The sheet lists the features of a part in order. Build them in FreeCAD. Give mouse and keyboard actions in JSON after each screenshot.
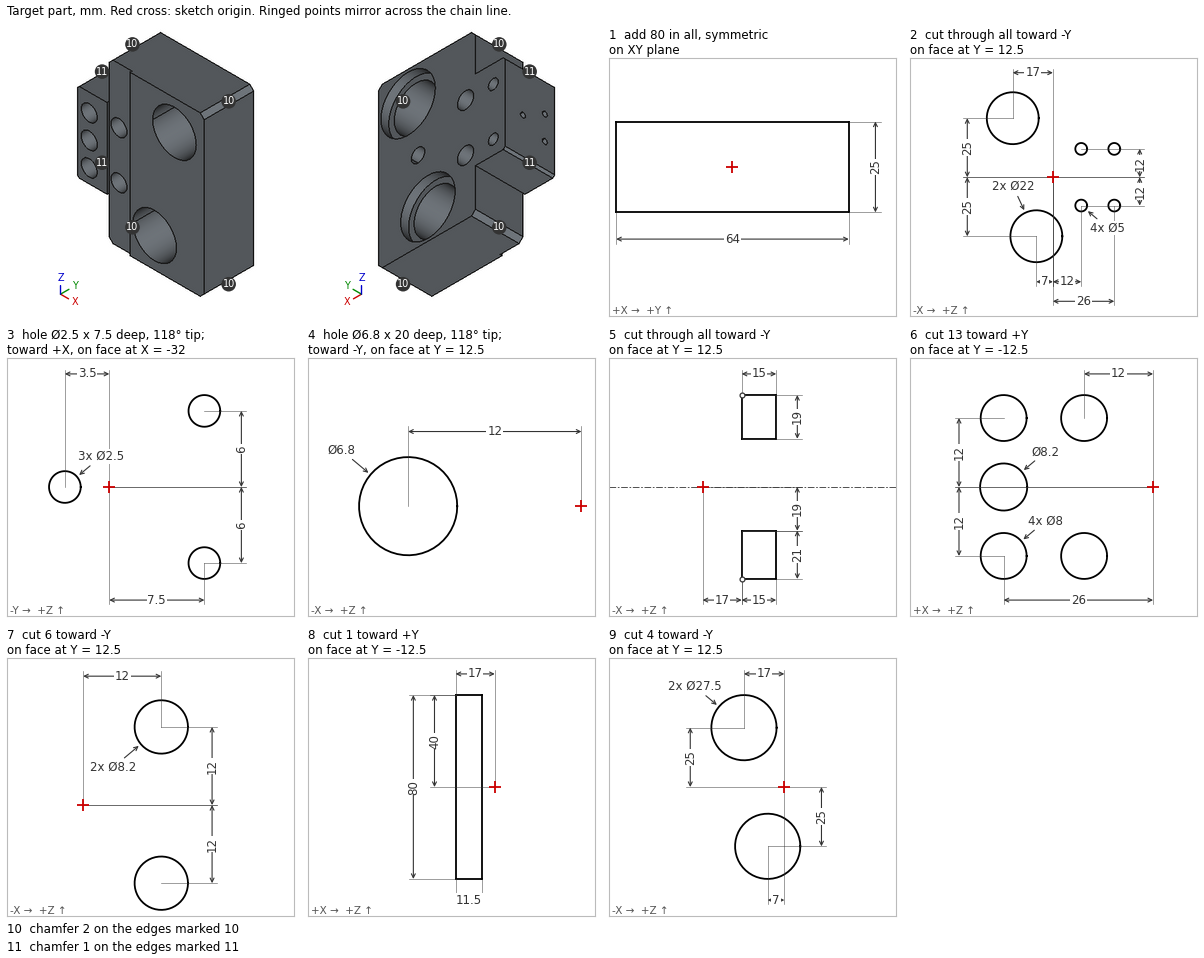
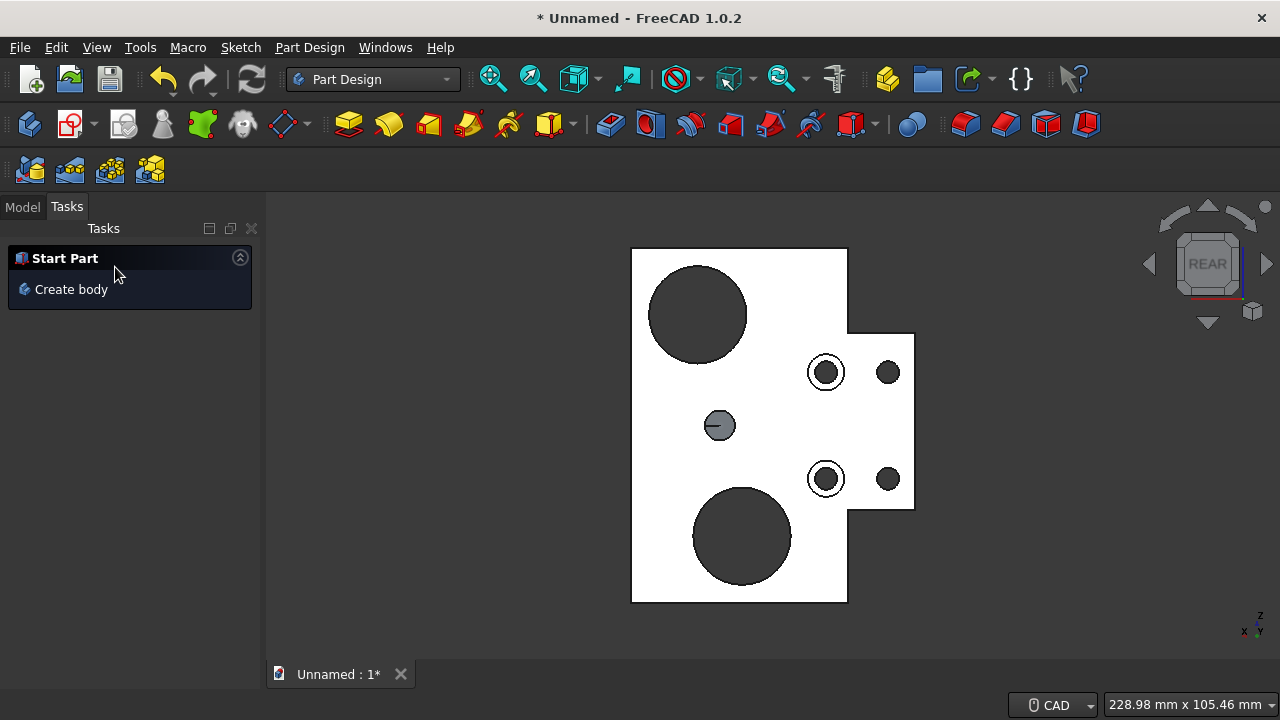
{"action": "key", "text": "0"}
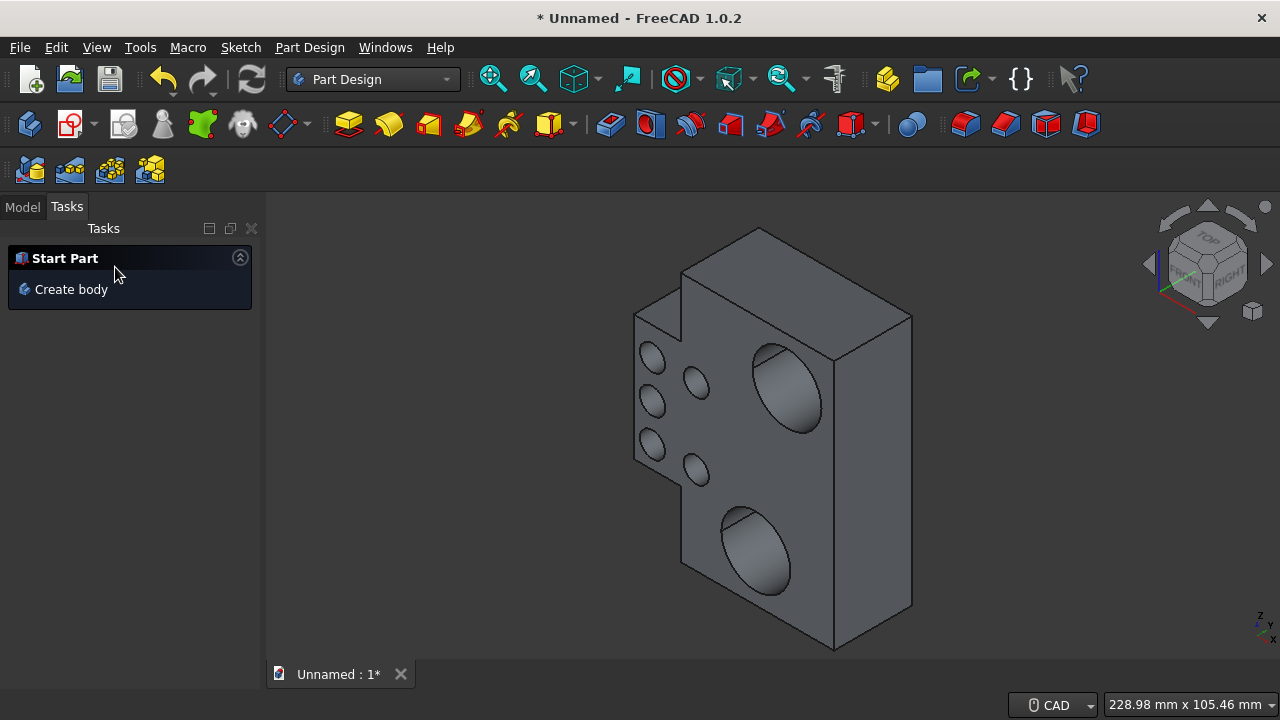
{"action": "left_click", "coordinate": [762, 464]}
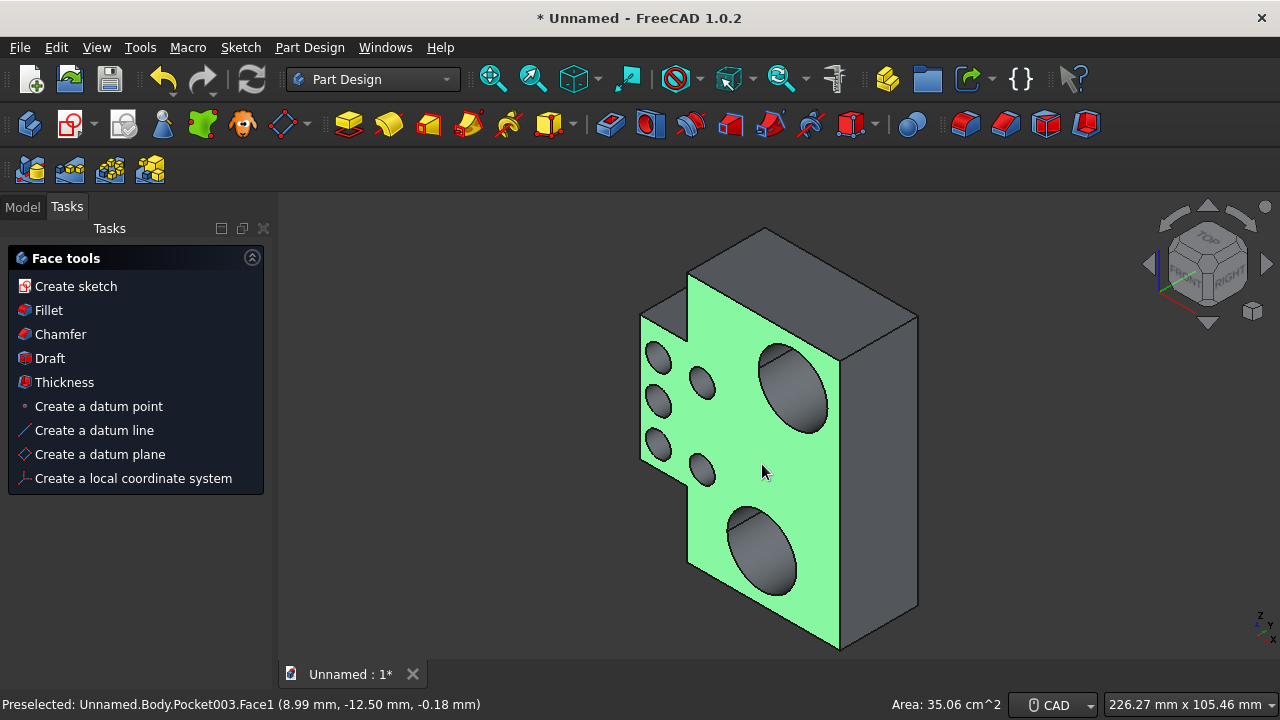
{"action": "left_click", "coordinate": [70, 124]}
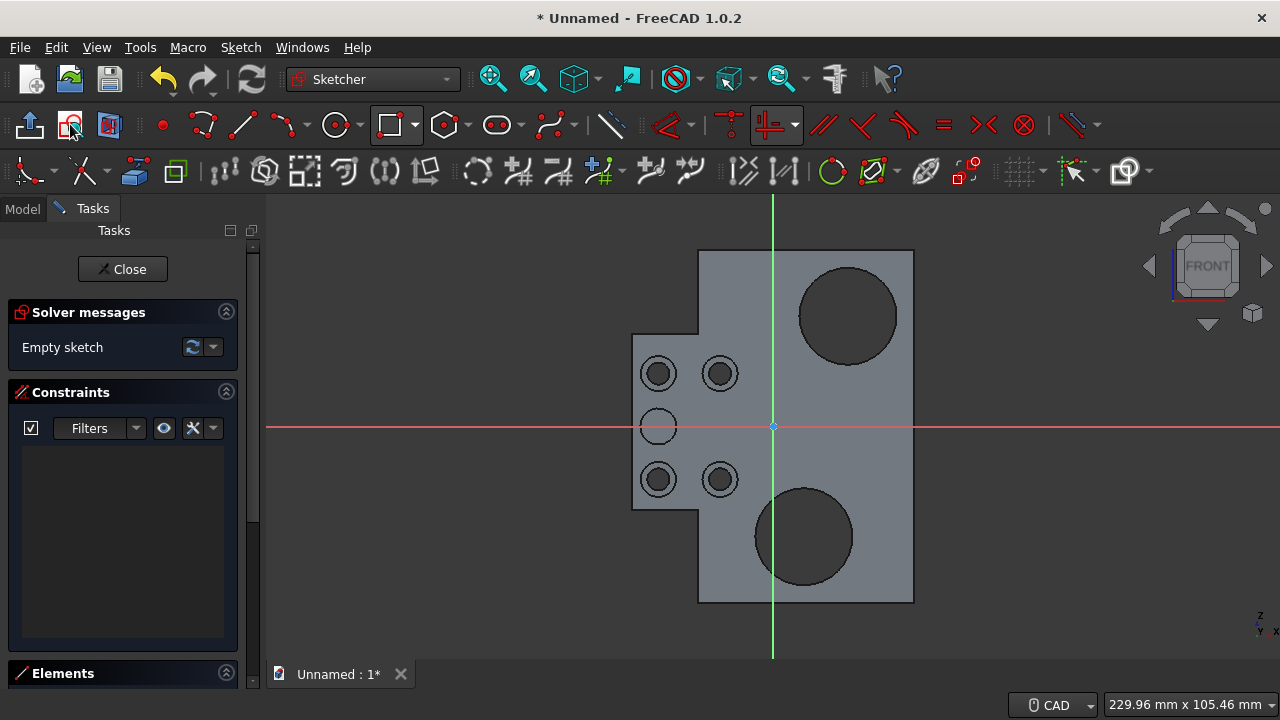
{"action": "left_click", "coordinate": [390, 126]}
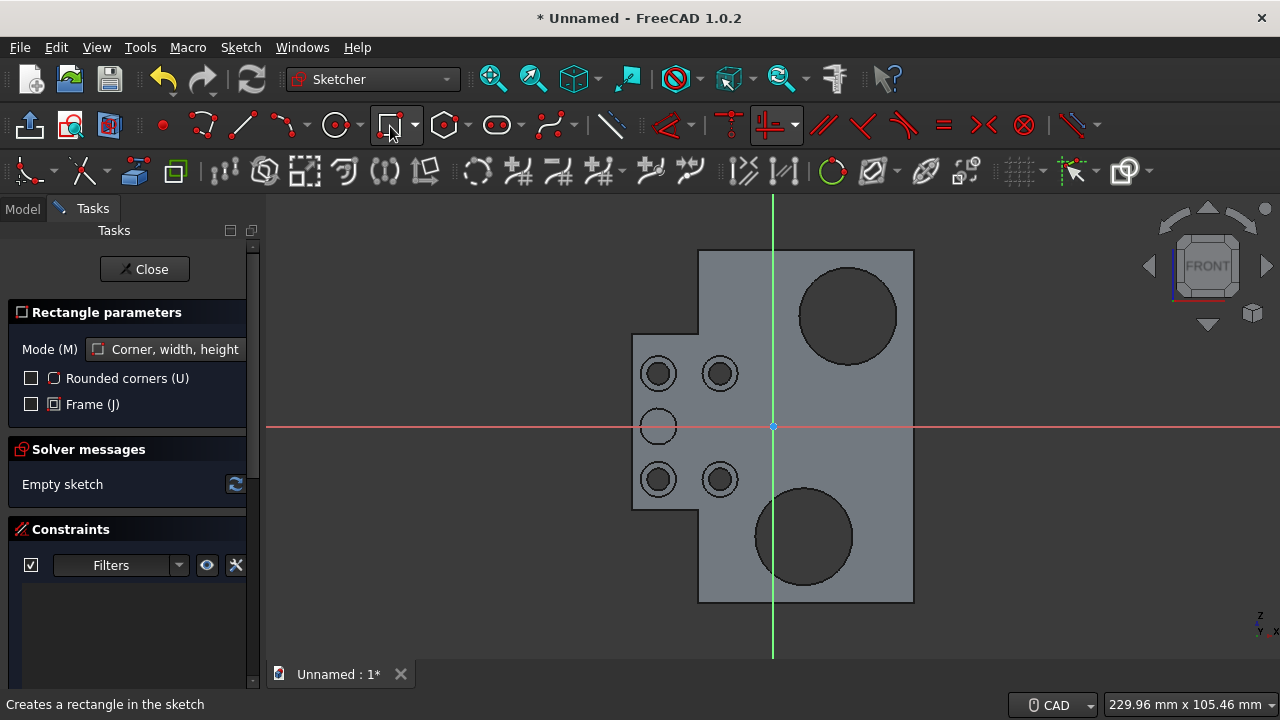
{"action": "left_click", "coordinate": [698, 250]}
{"action": "left_click", "coordinate": [749, 603]}
{"action": "key", "text": "Escape"}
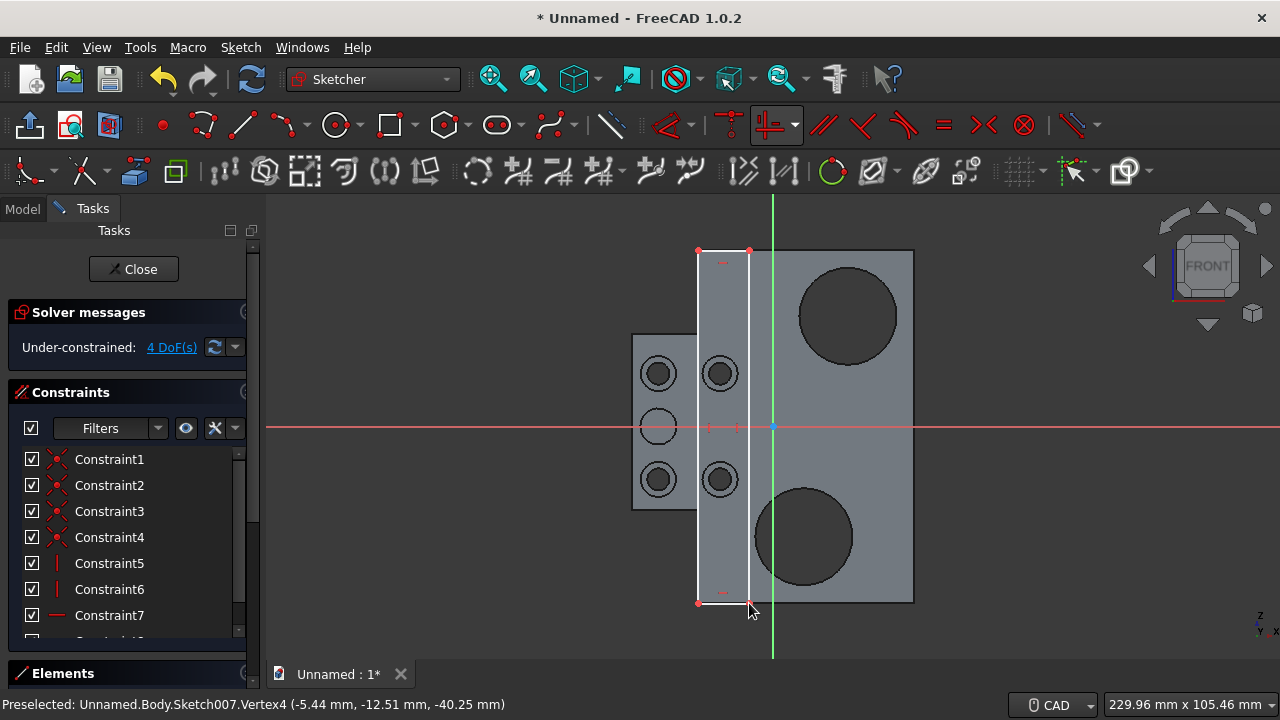
{"action": "left_click", "coordinate": [666, 126]}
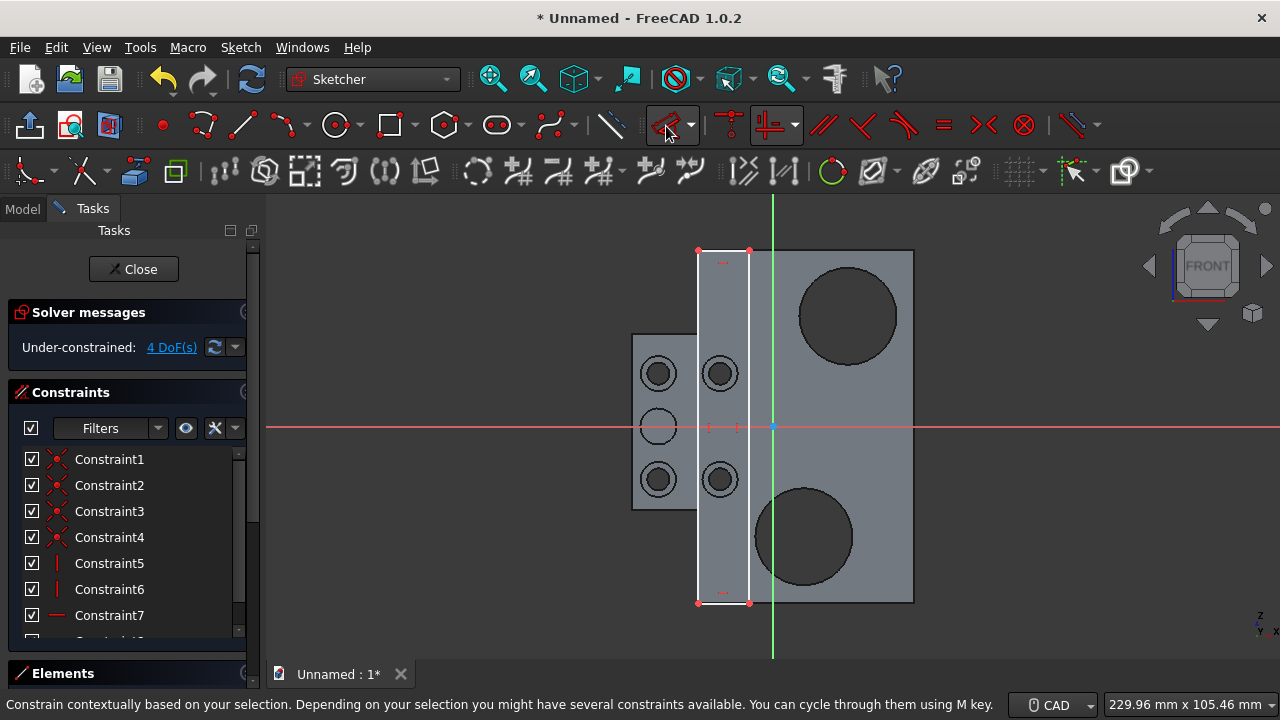
{"action": "left_click", "coordinate": [698, 357]}
{"action": "left_click", "coordinate": [664, 346]}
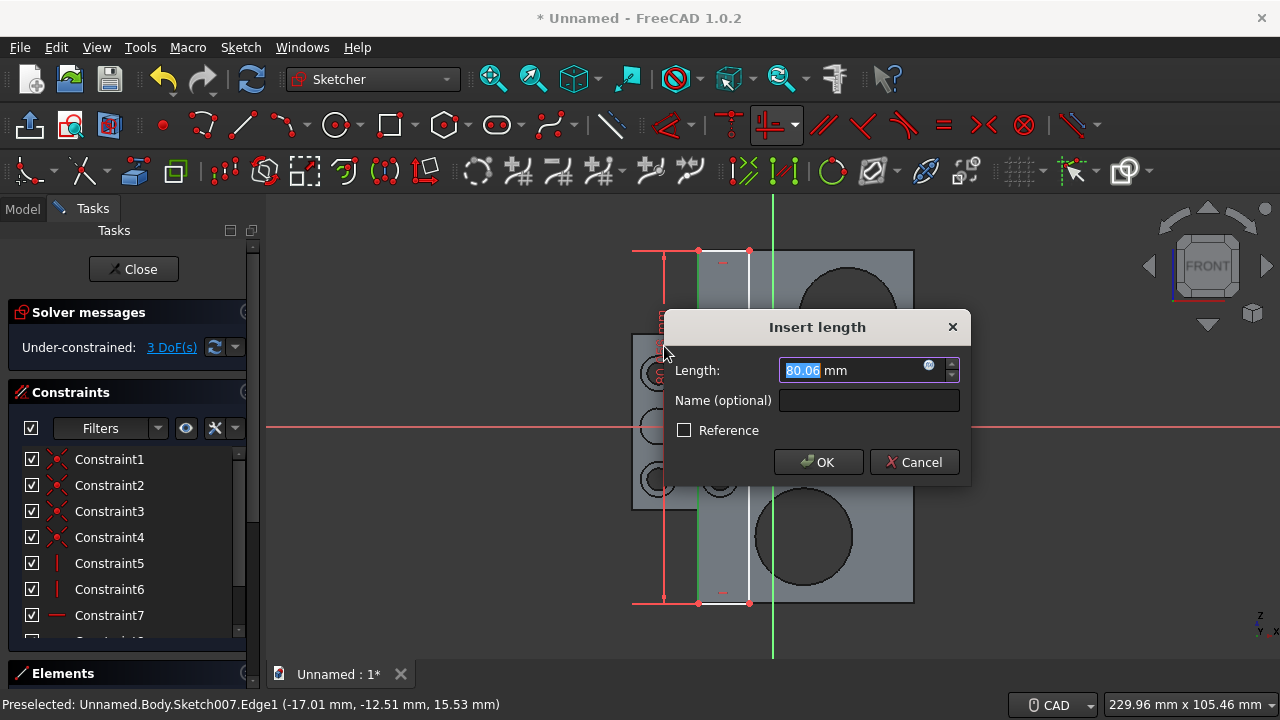
{"action": "type", "text": "80"}
{"action": "key", "text": "Return"}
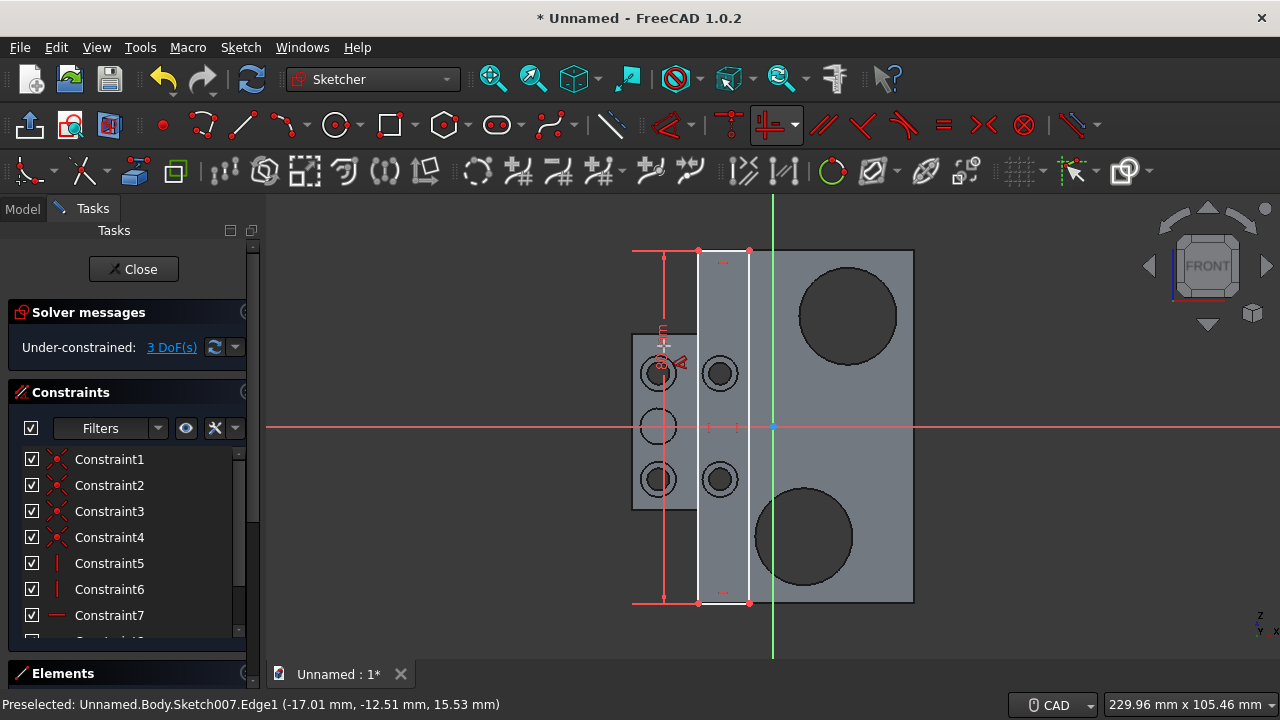
{"action": "left_click", "coordinate": [698, 251]}
{"action": "left_click", "coordinate": [735, 461]}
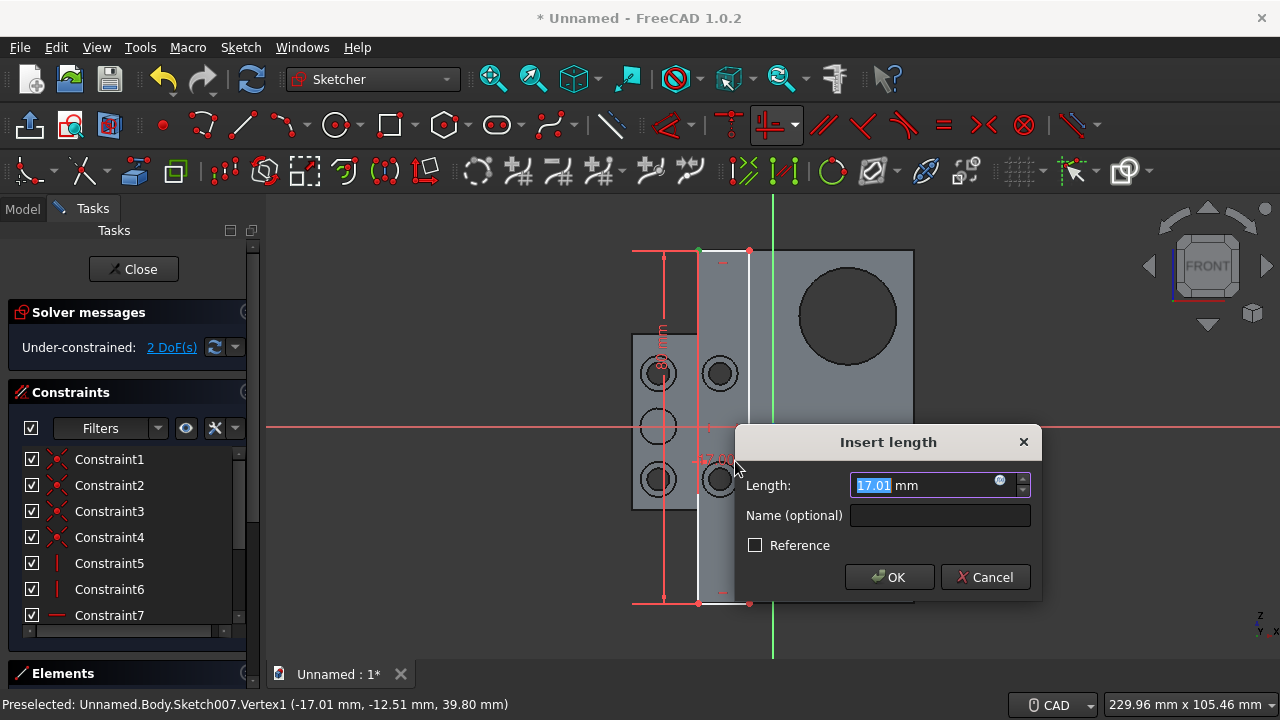
{"action": "type", "text": "17"}
{"action": "key", "text": "Return"}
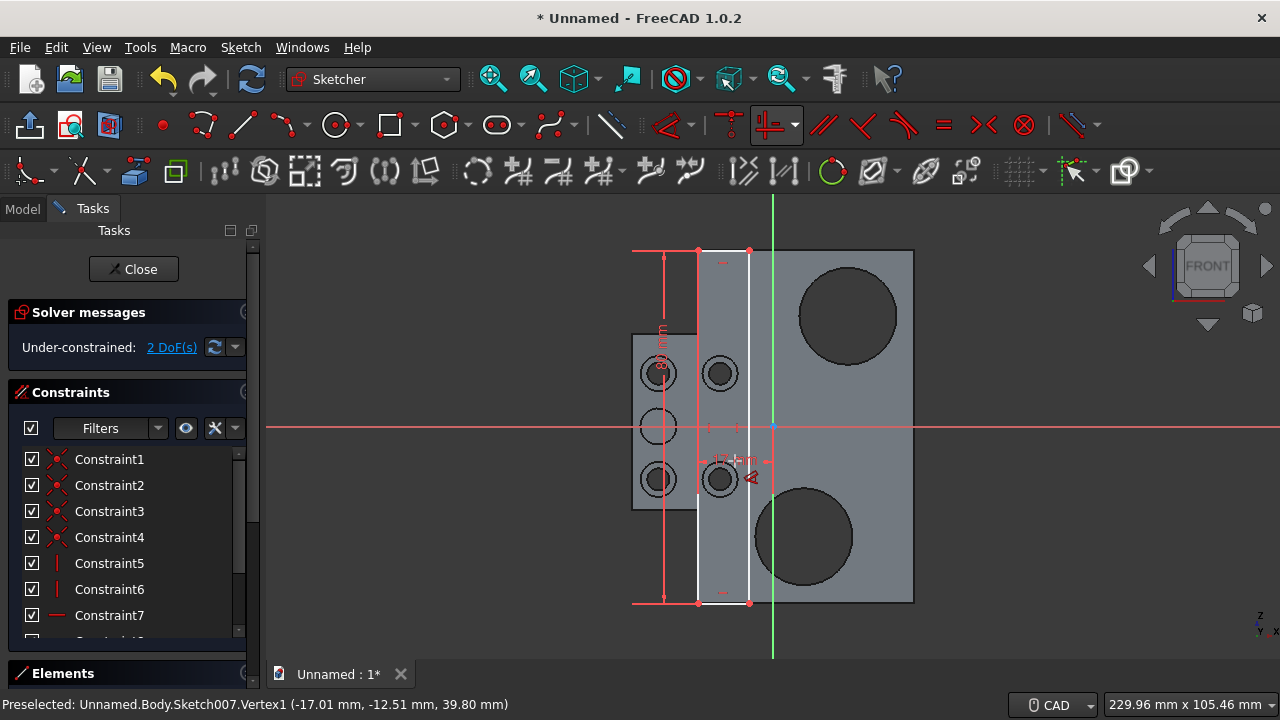
{"action": "left_click", "coordinate": [698, 251]}
{"action": "left_click", "coordinate": [807, 339]}